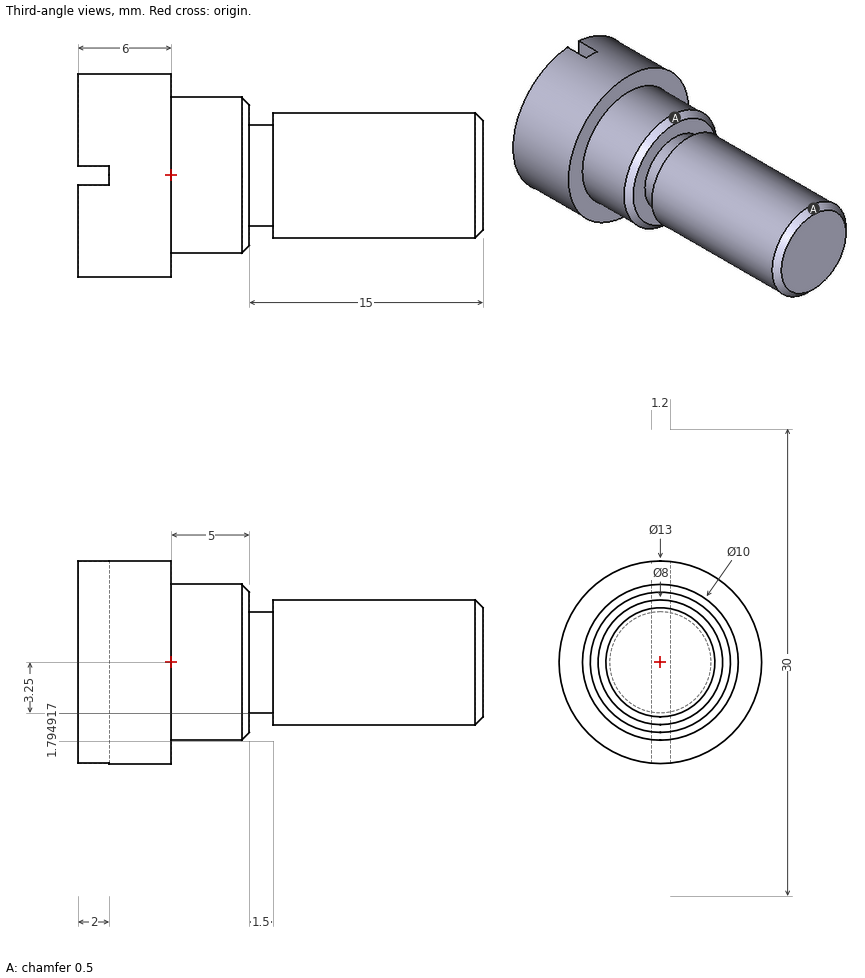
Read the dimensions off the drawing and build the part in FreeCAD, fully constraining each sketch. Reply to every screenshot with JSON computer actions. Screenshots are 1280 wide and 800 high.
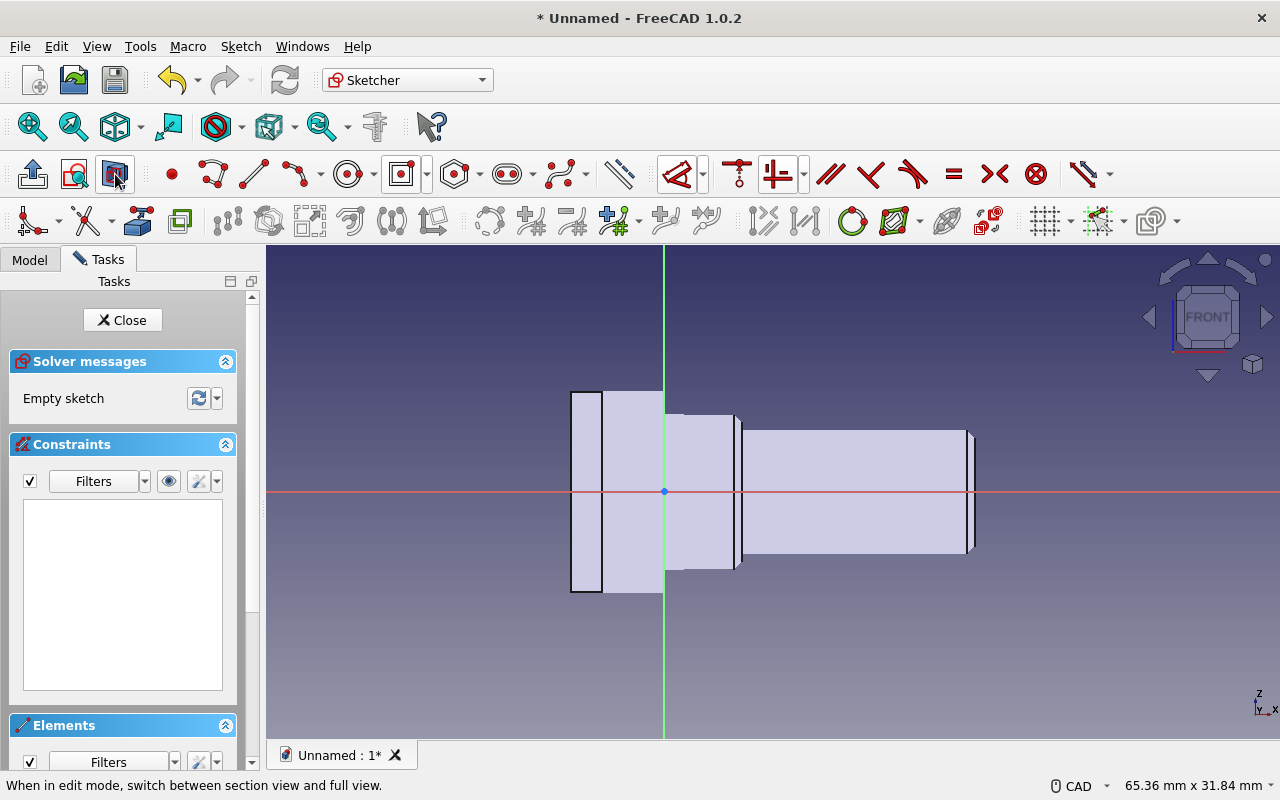
{"action": "scroll", "coordinate": [759, 563], "scroll_direction": "up", "scroll_amount": 12}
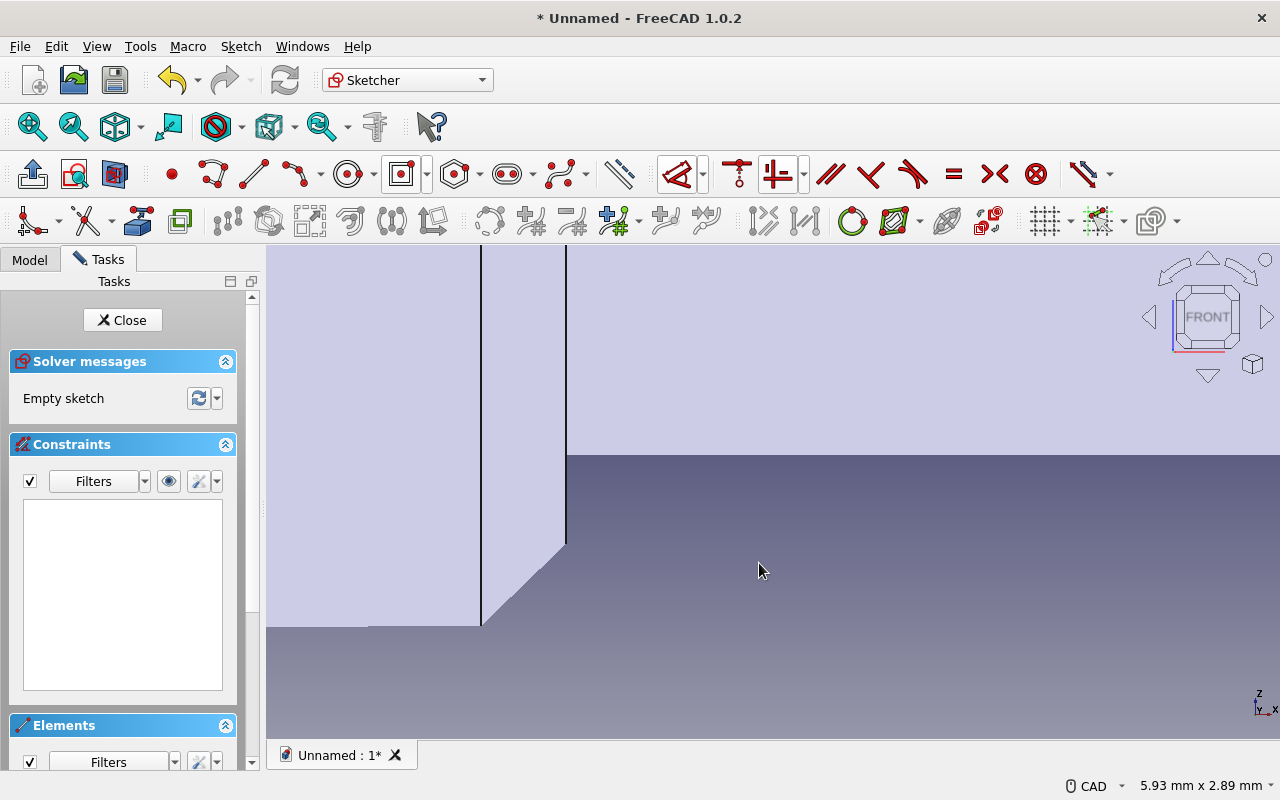
{"action": "key", "text": "g r"}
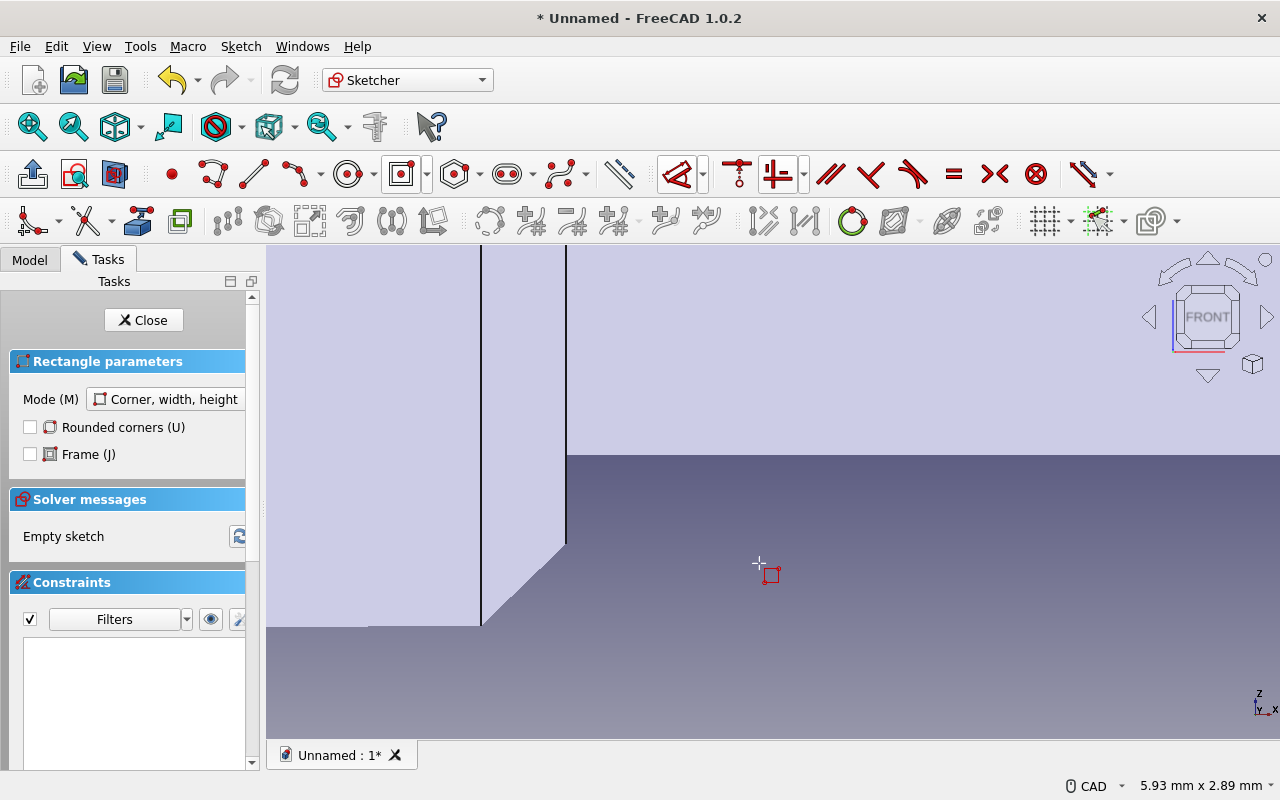
{"action": "left_click", "coordinate": [566, 330]}
{"action": "mouse_move", "coordinate": [823, 637]}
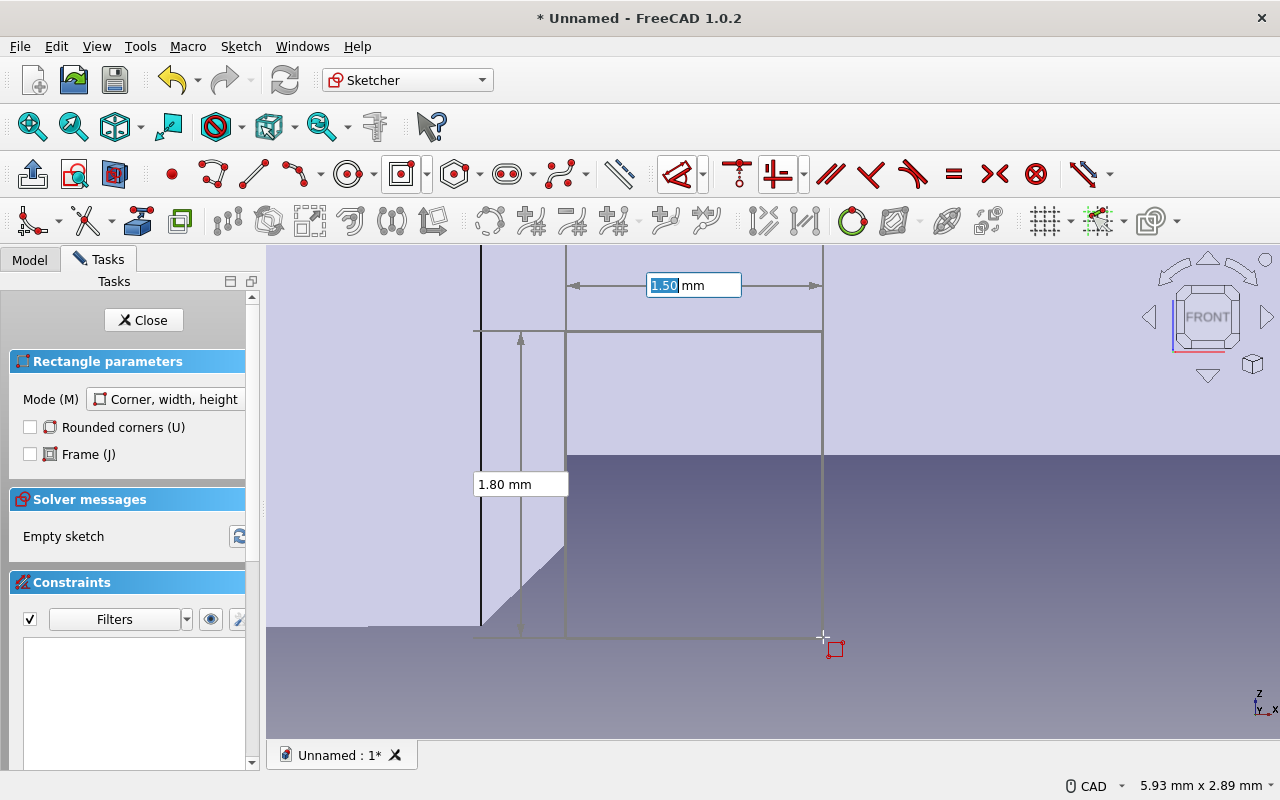
{"action": "type", "text": "1.5"}
{"action": "key", "text": "Tab"}
{"action": "type", "text": "1.794917"}
{"action": "key", "text": "Return"}
{"action": "key", "text": "Escape"}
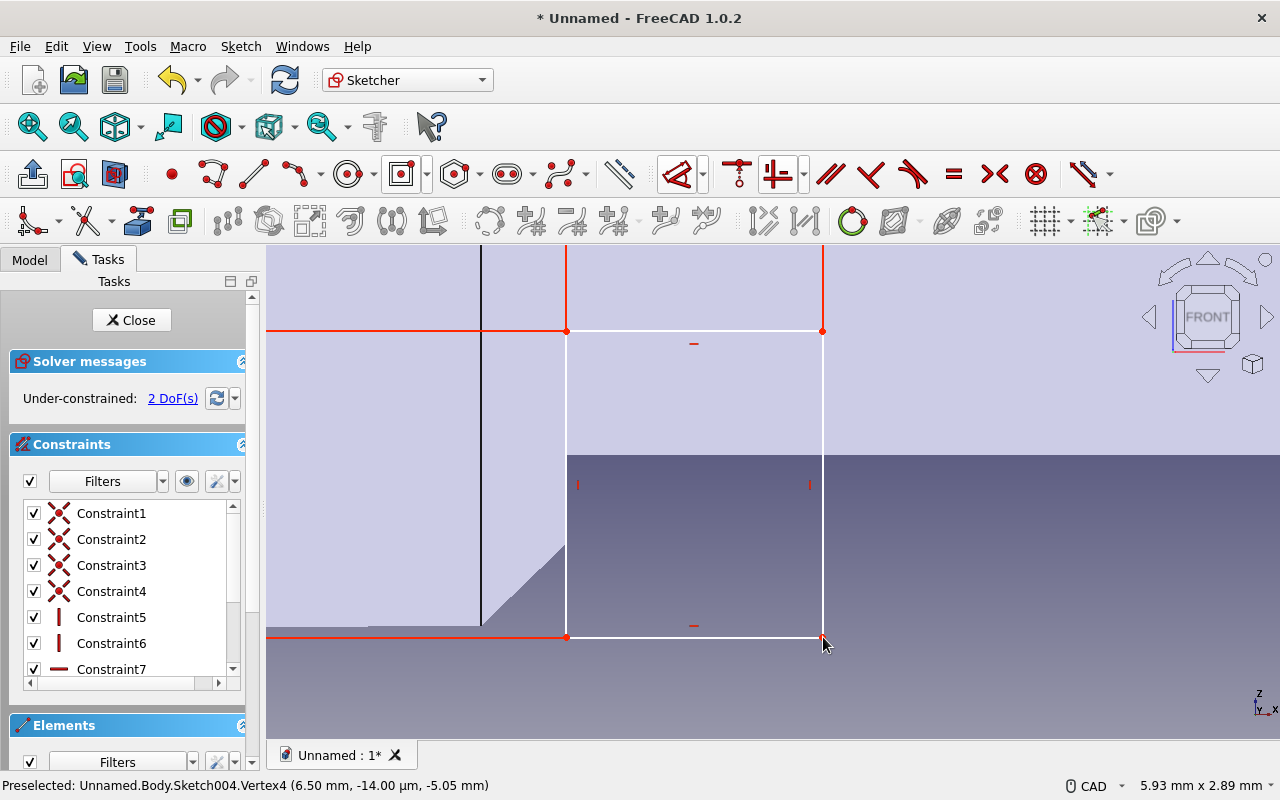
{"action": "left_click", "coordinate": [676, 174]}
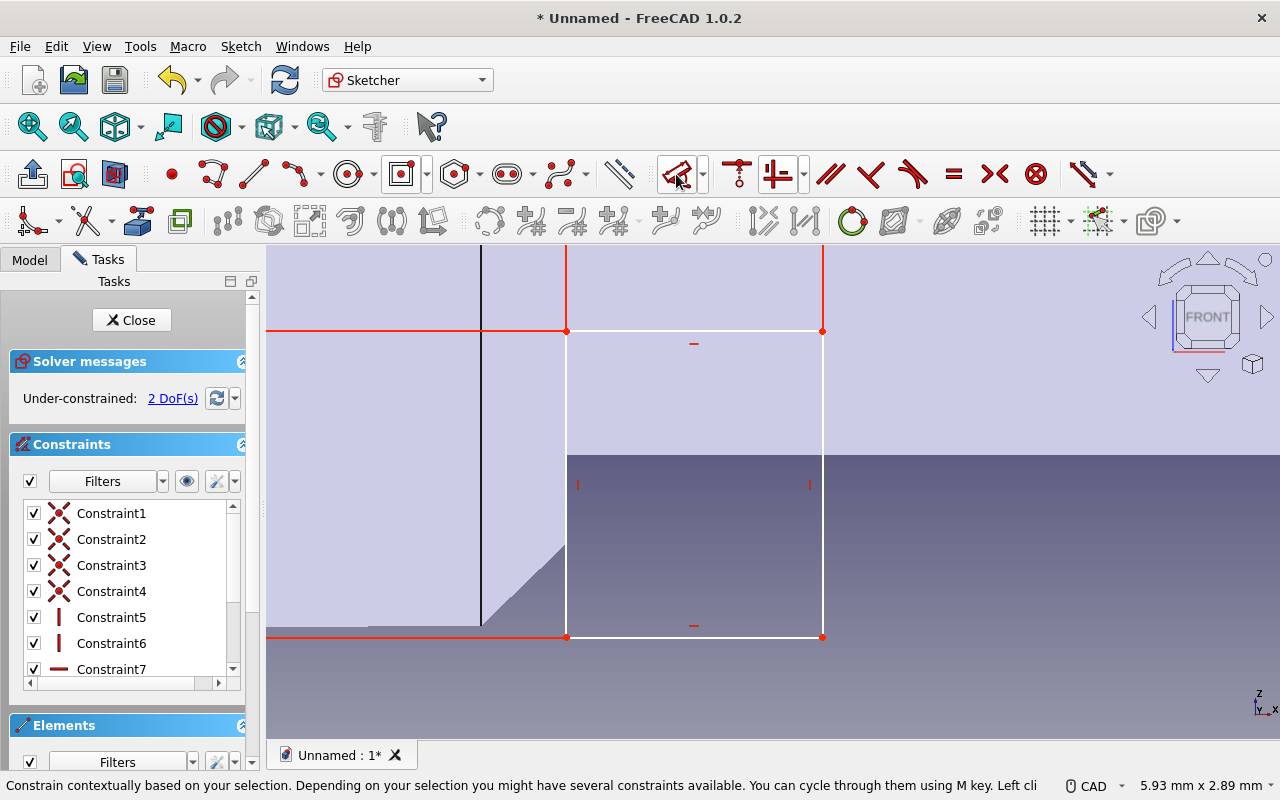
{"action": "left_click", "coordinate": [566, 331]}
{"action": "left_click", "coordinate": [430, 365]}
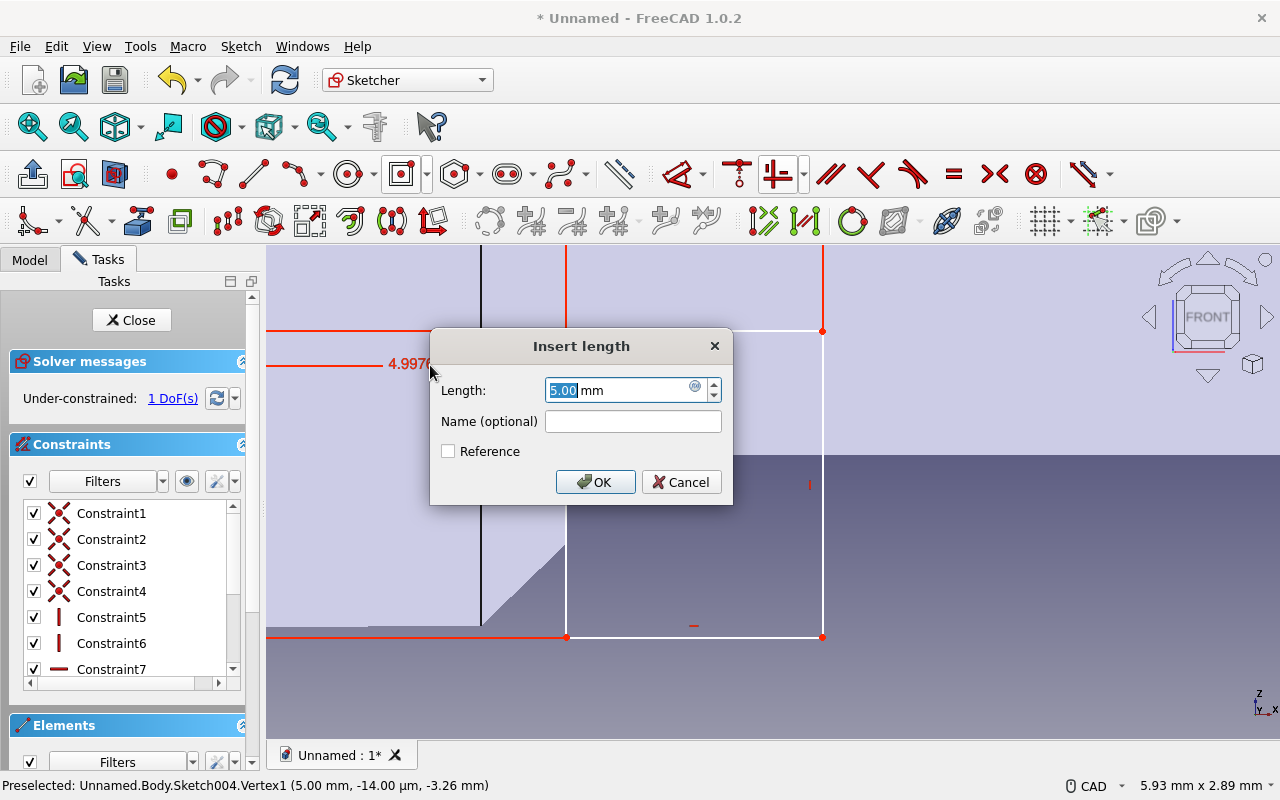
{"action": "type", "text": "5"}
{"action": "key", "text": "Return"}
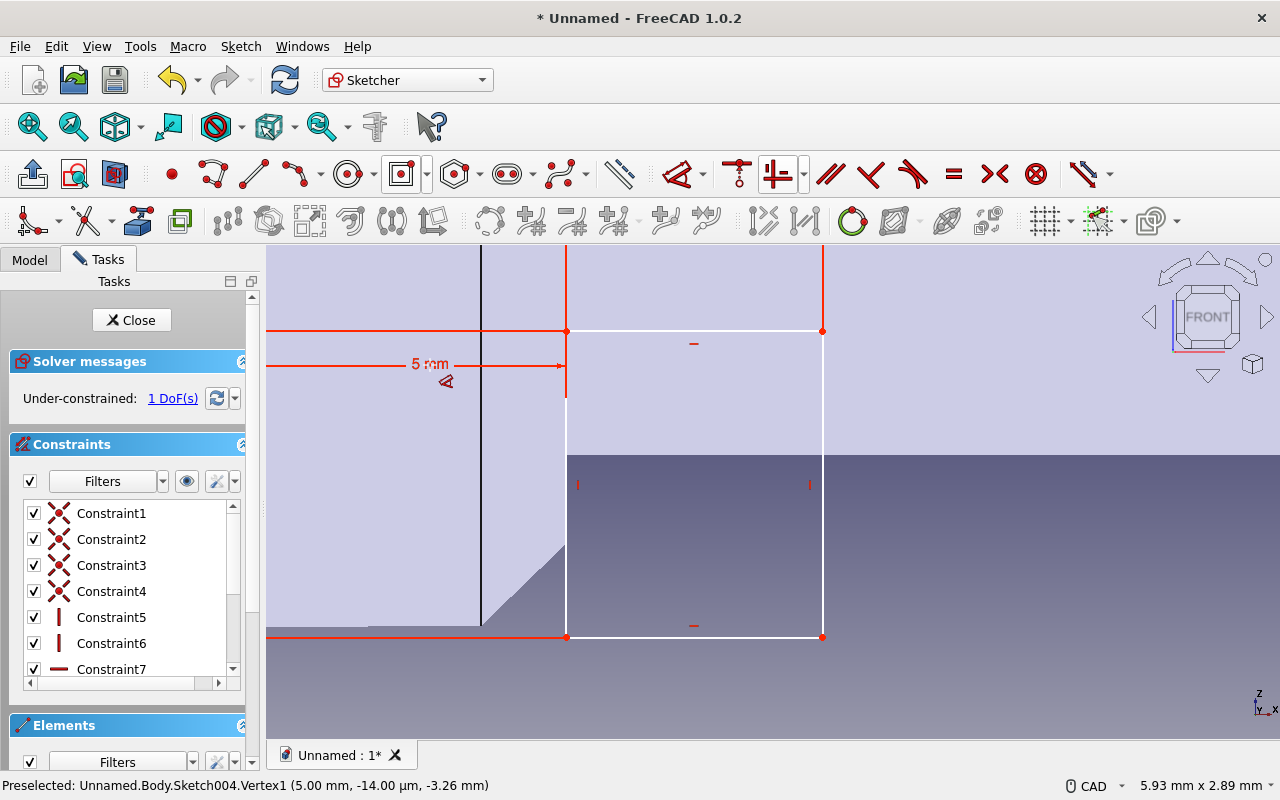
{"action": "left_click", "coordinate": [566, 331]}
{"action": "left_click", "coordinate": [600, 302]}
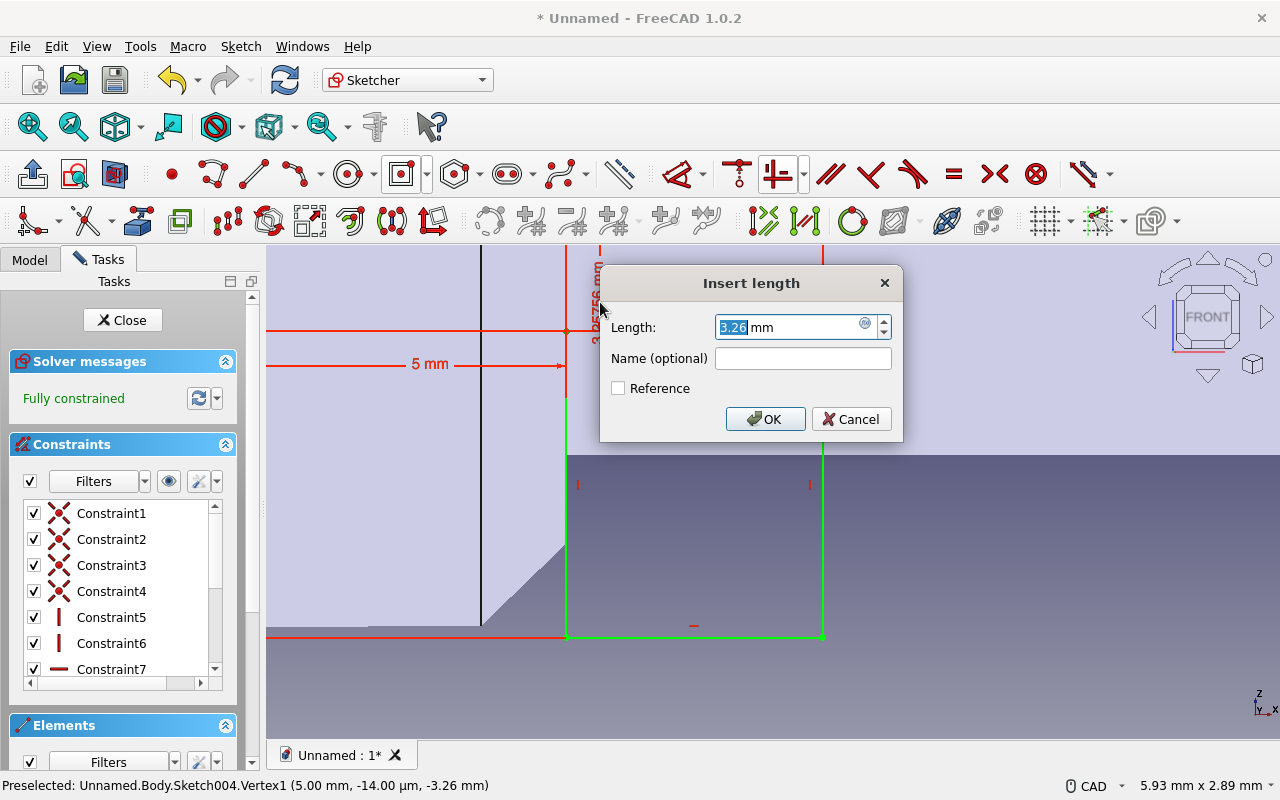
{"action": "type", "text": "3.25"}
{"action": "key", "text": "Return"}
{"action": "key", "text": "Escape"}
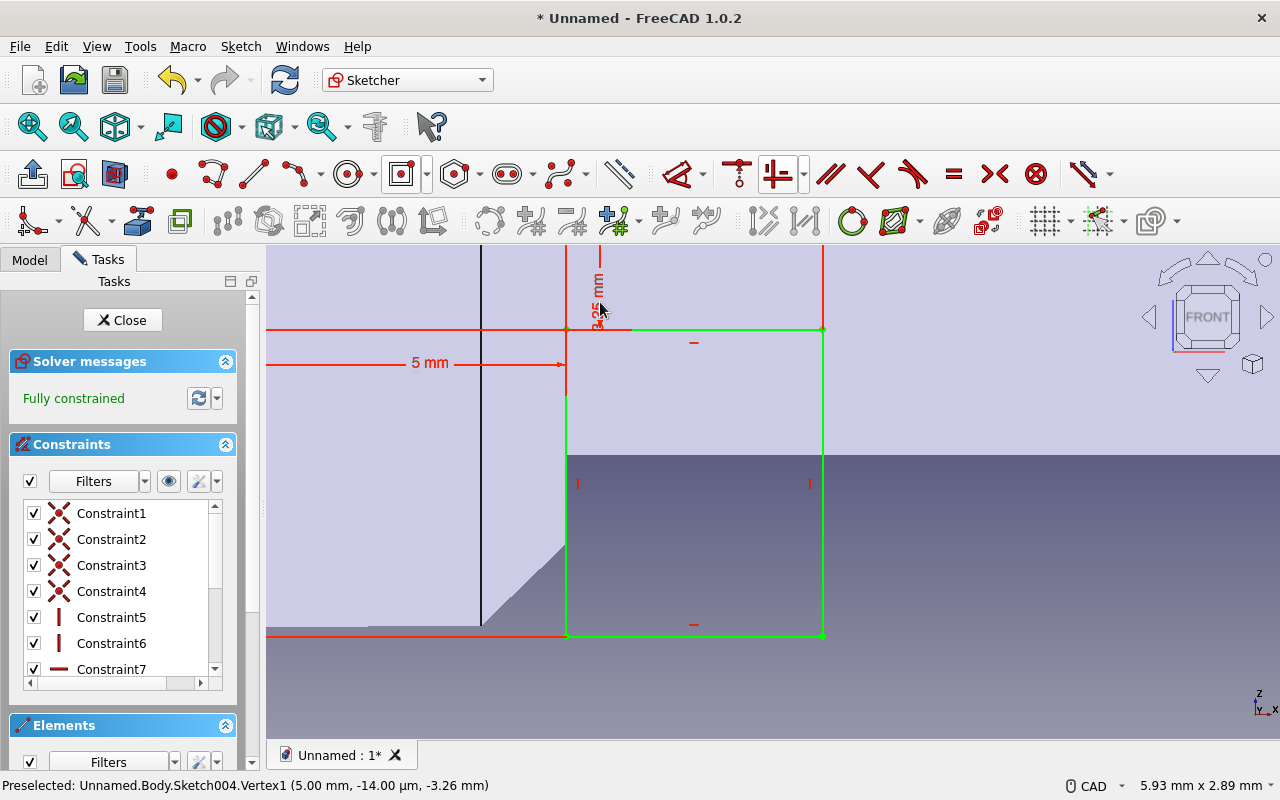
{"action": "left_click", "coordinate": [123, 320]}